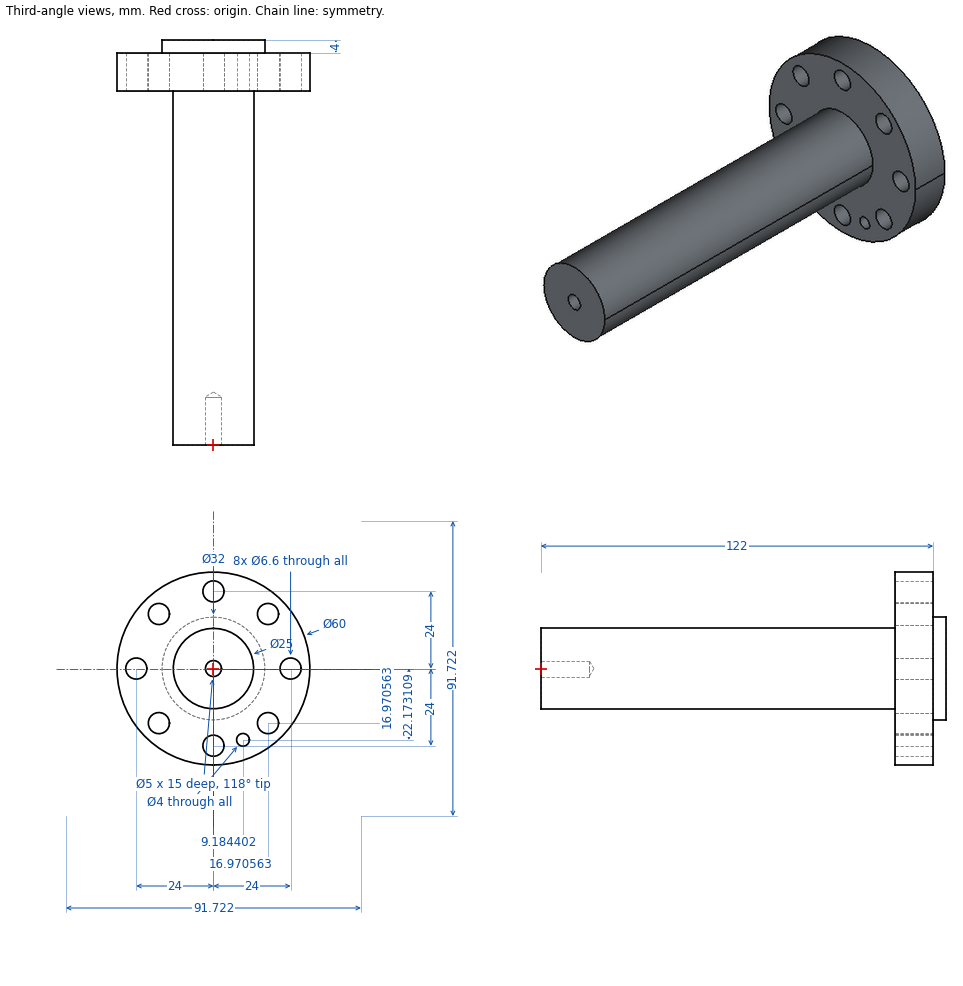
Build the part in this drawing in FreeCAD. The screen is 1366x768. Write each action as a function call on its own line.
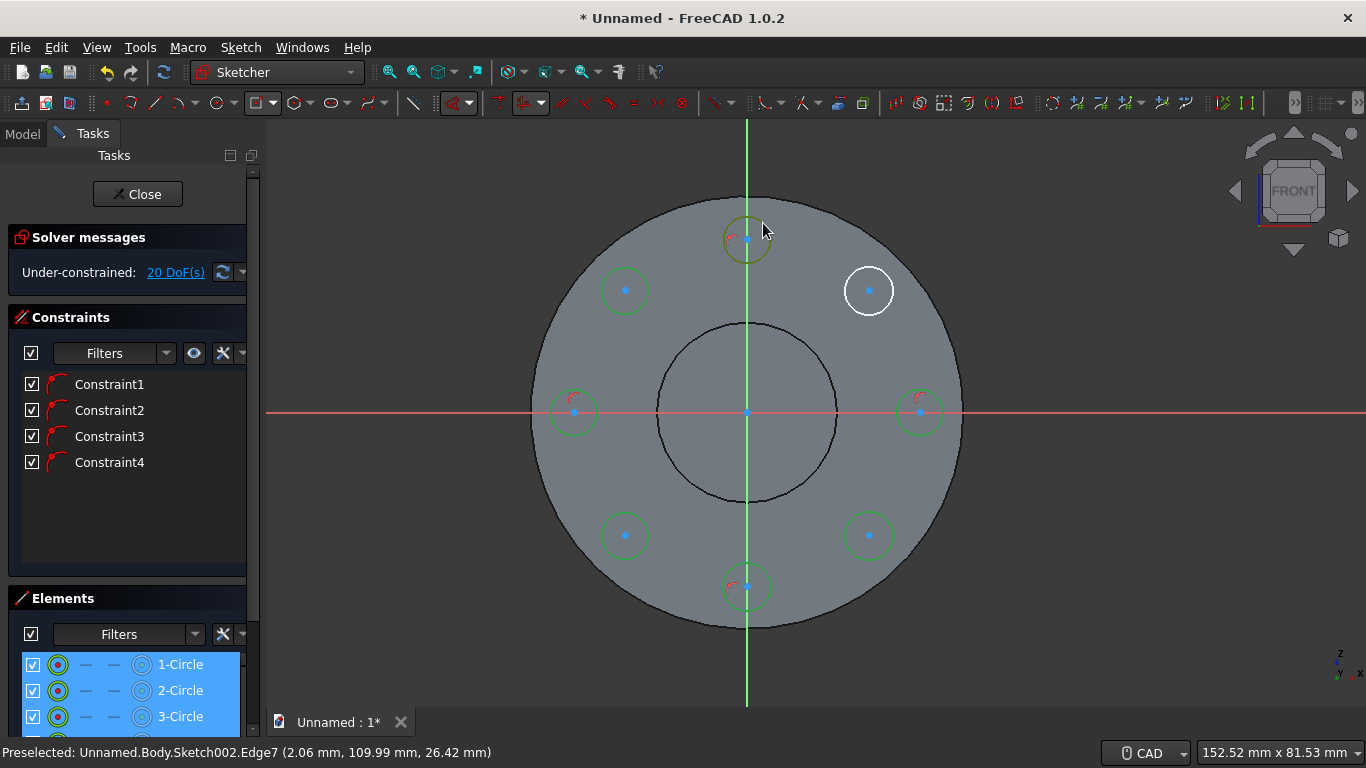
click(886, 274)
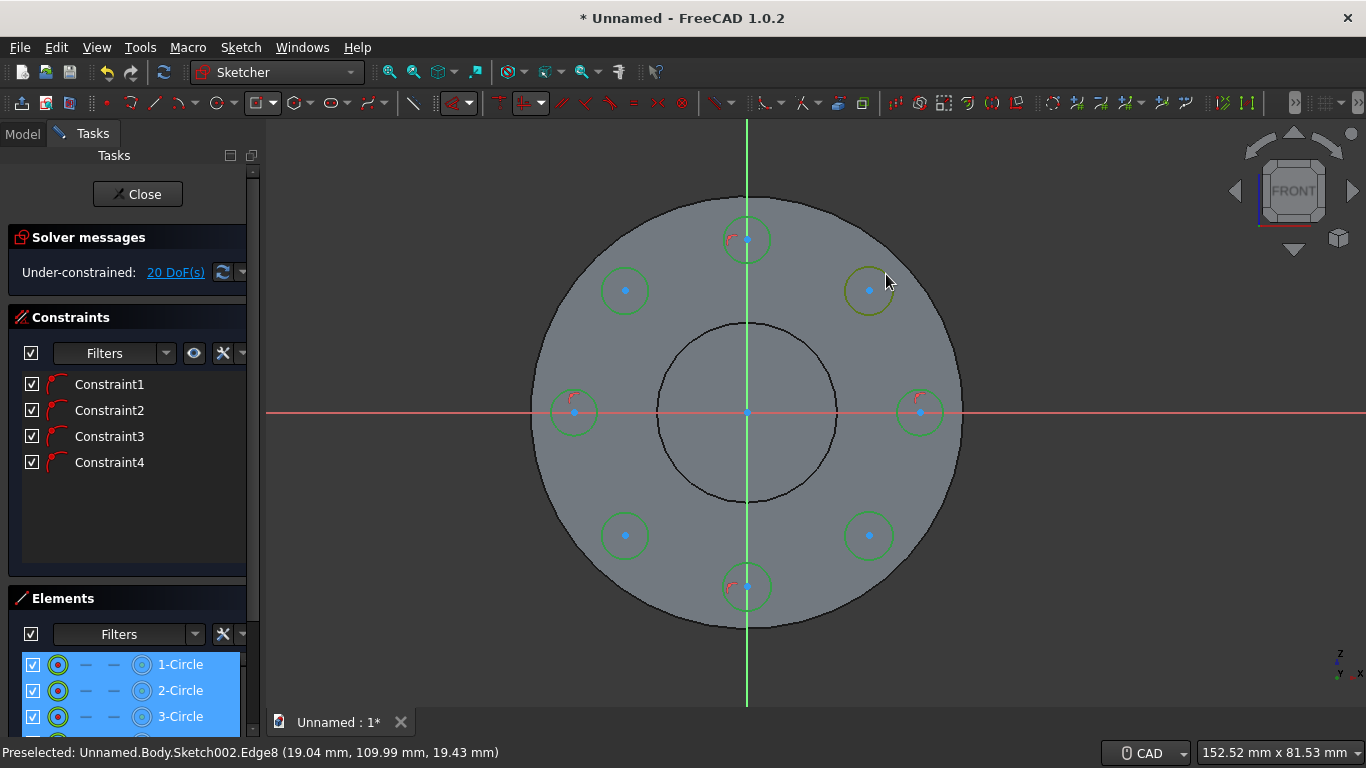
click(634, 104)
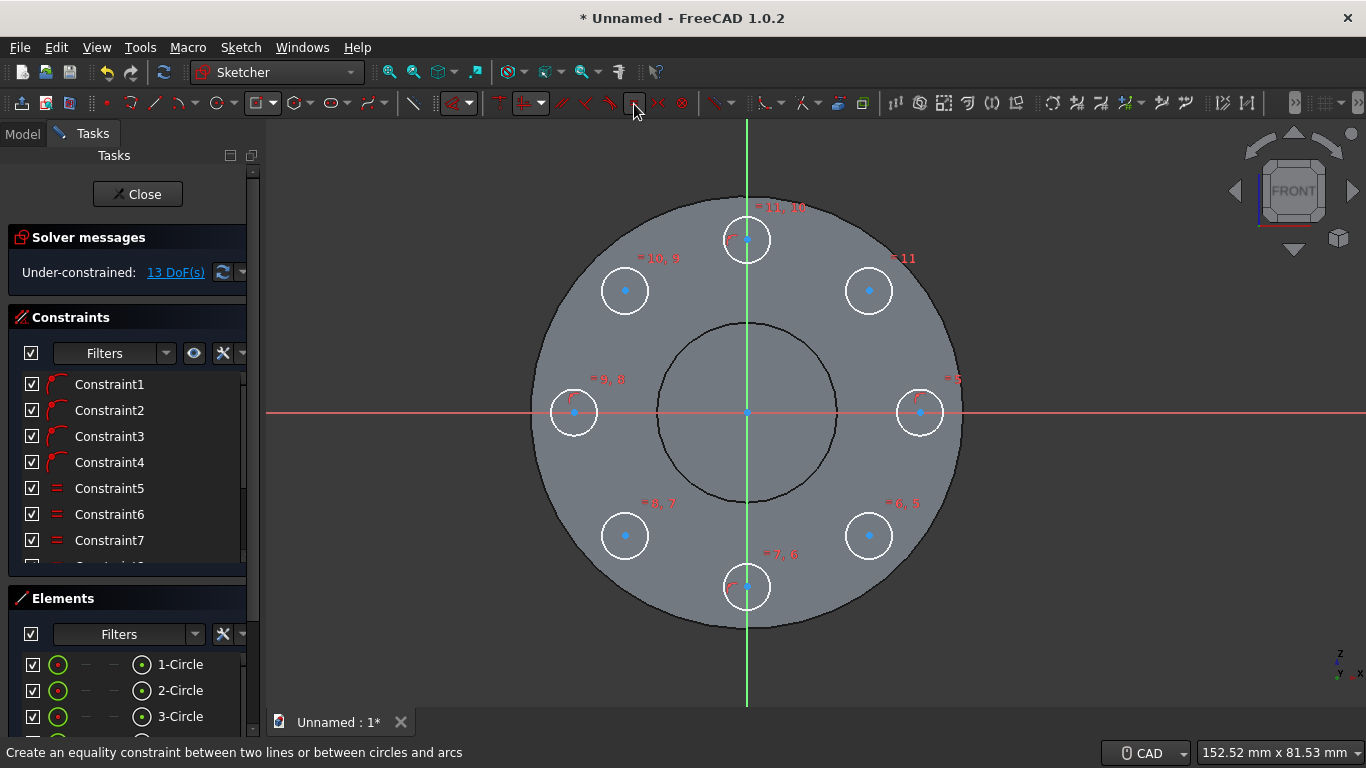
click(869, 536)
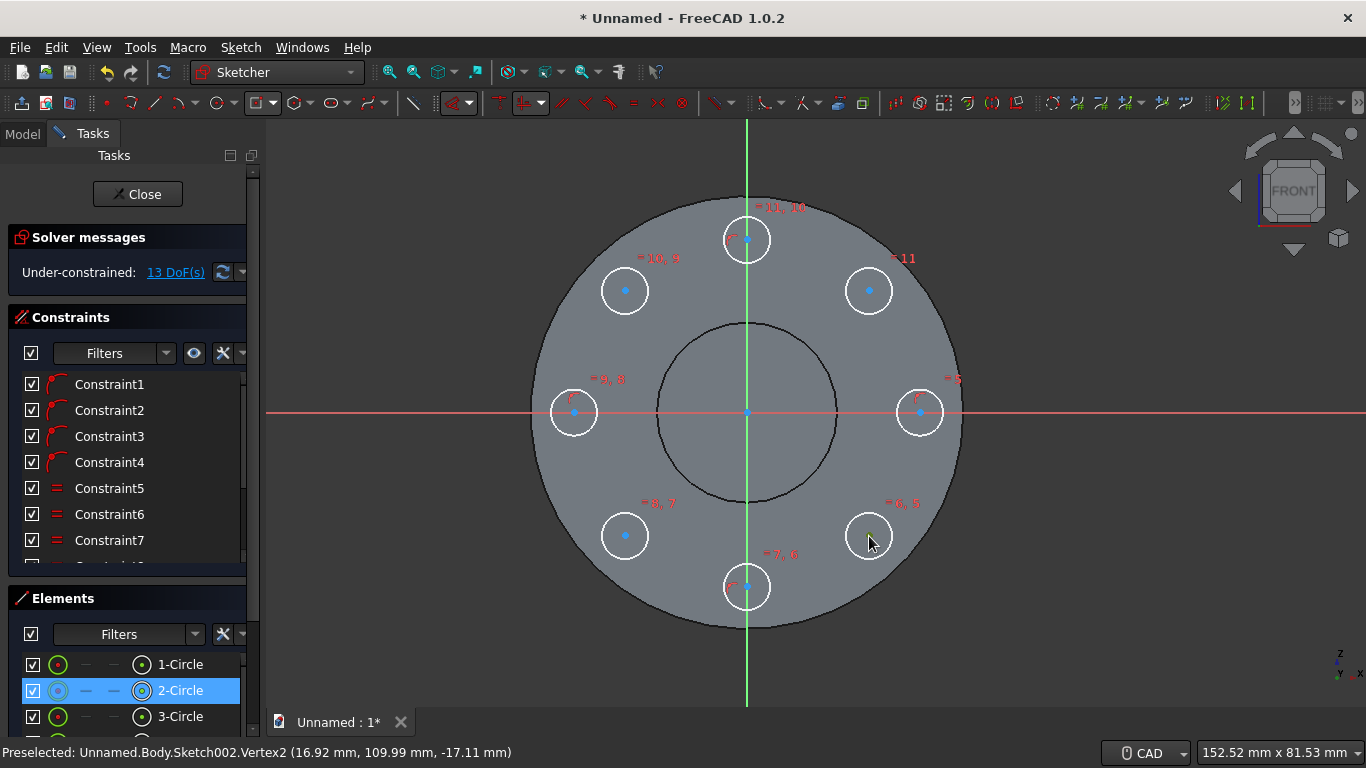
click(625, 536)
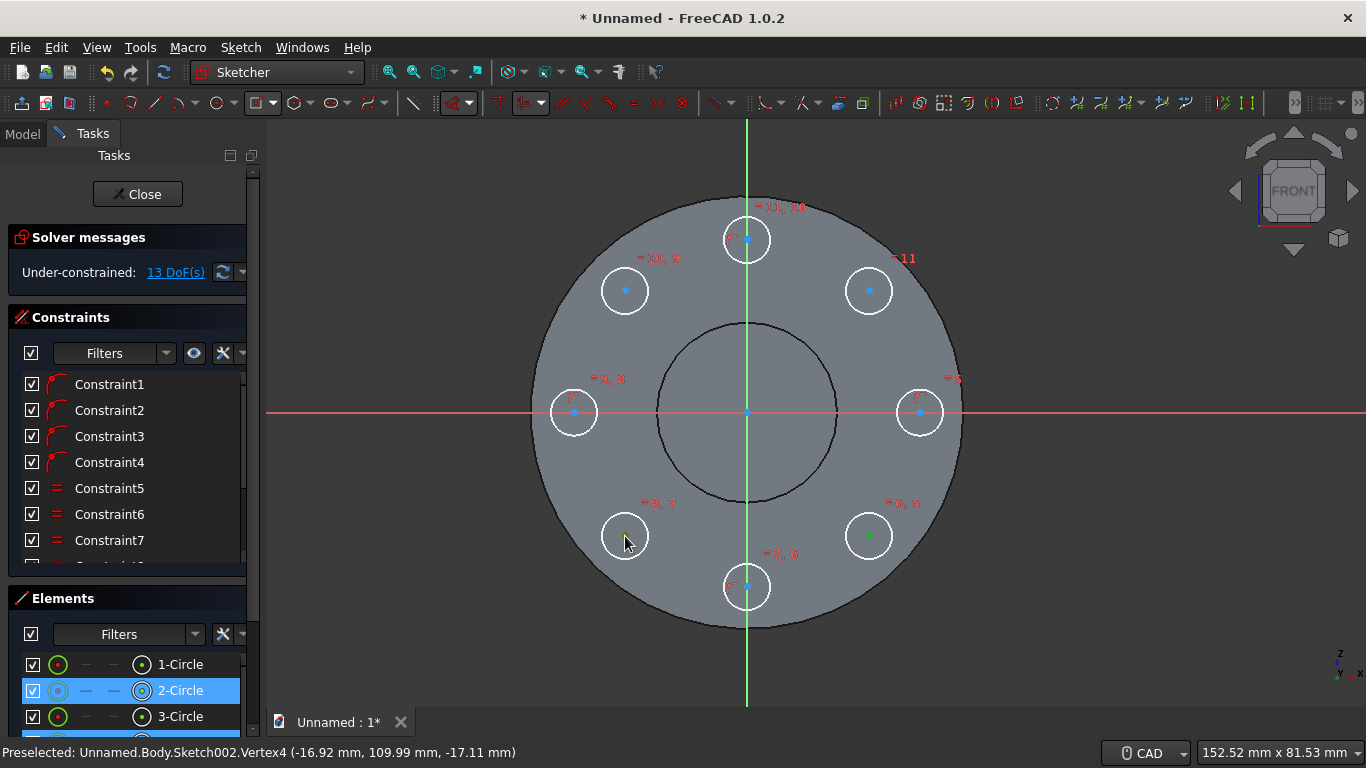
click(747, 641)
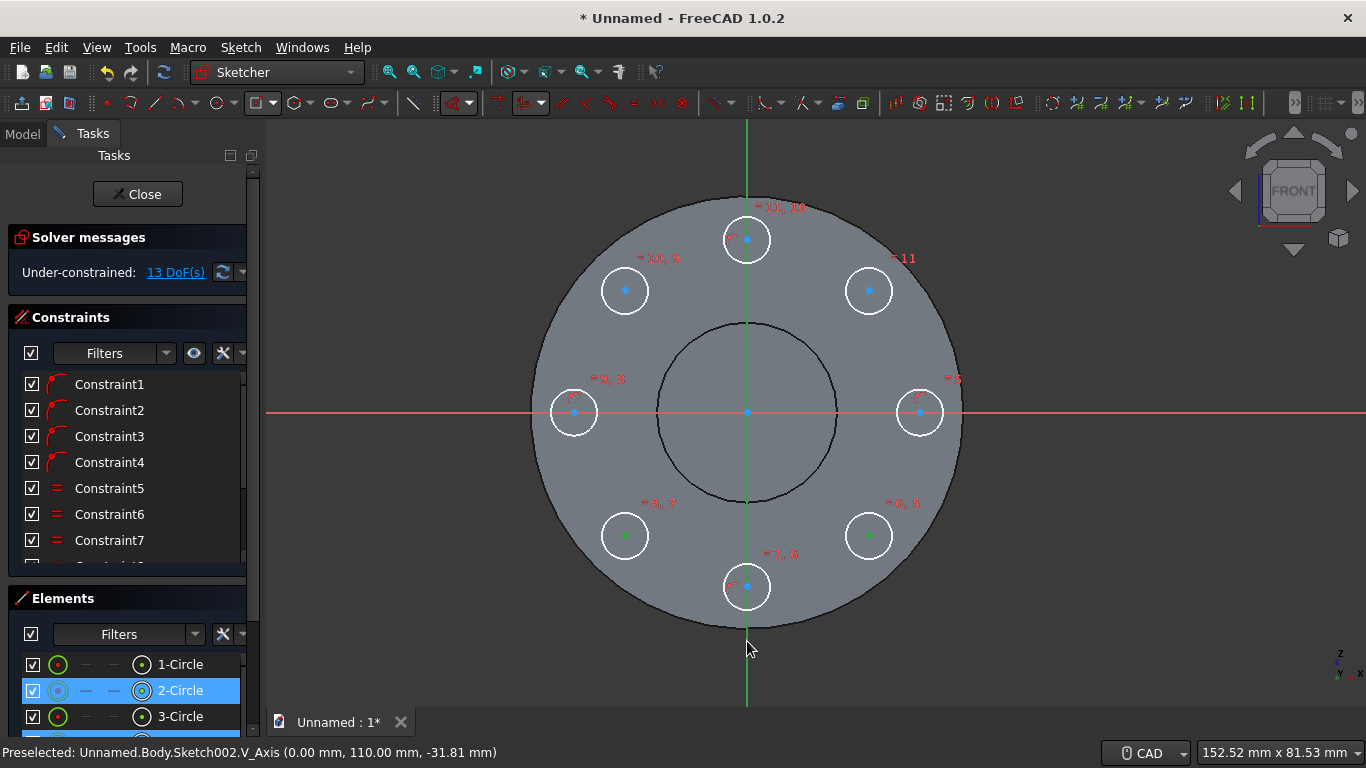
key(s)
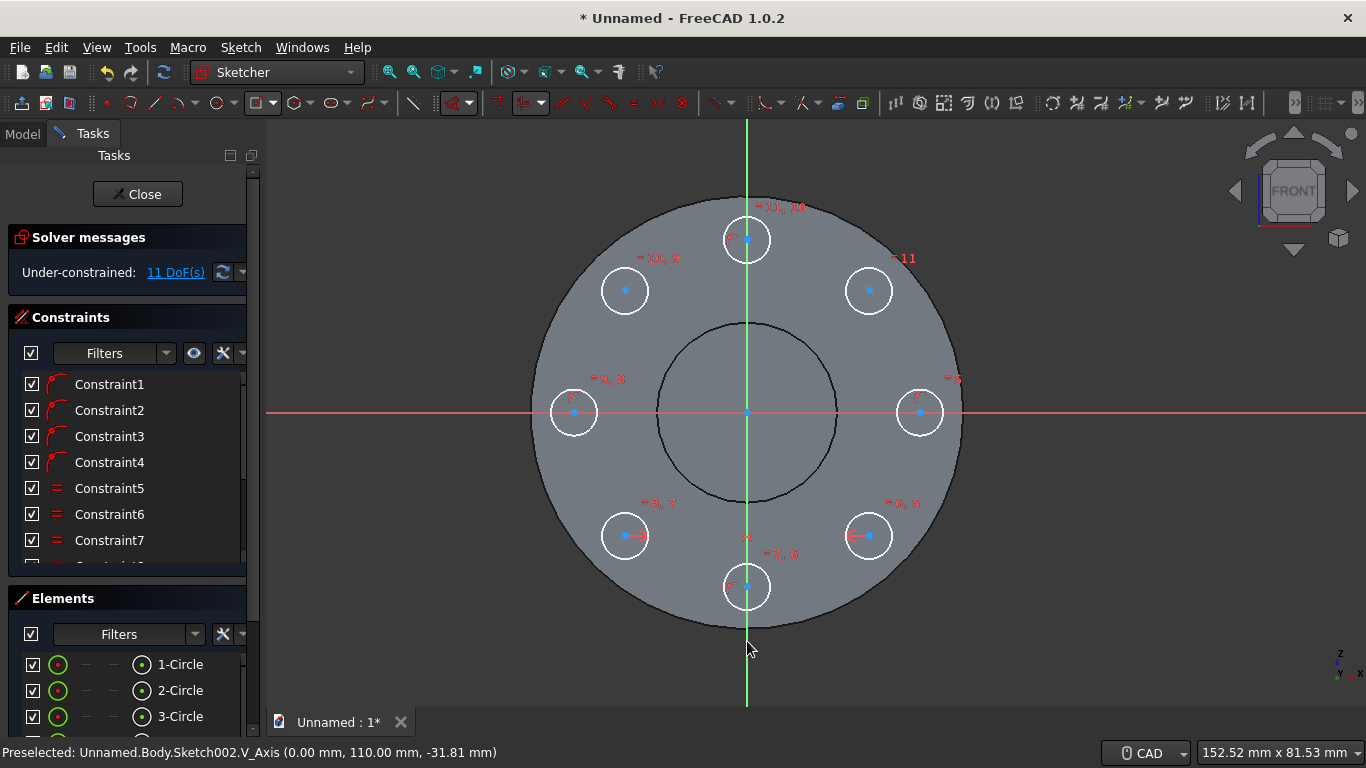
click(625, 536)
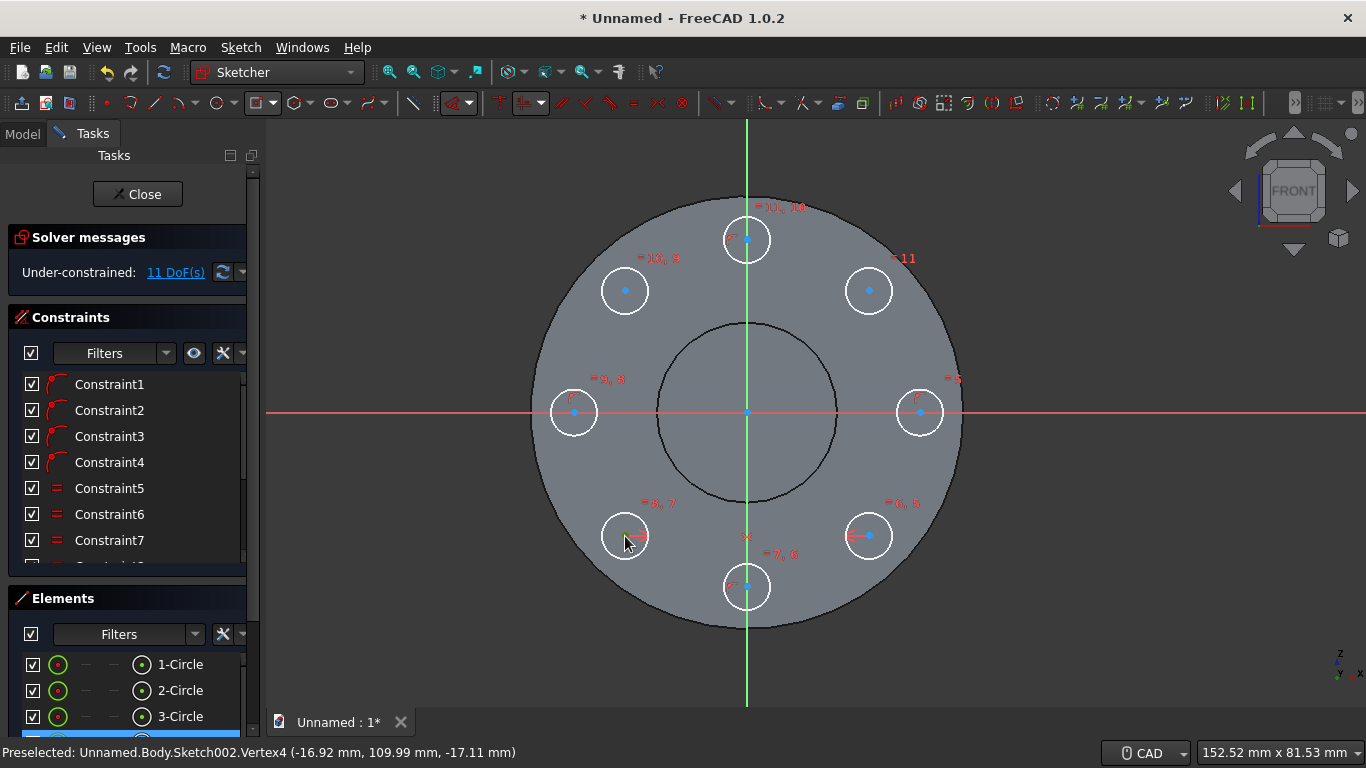
click(625, 291)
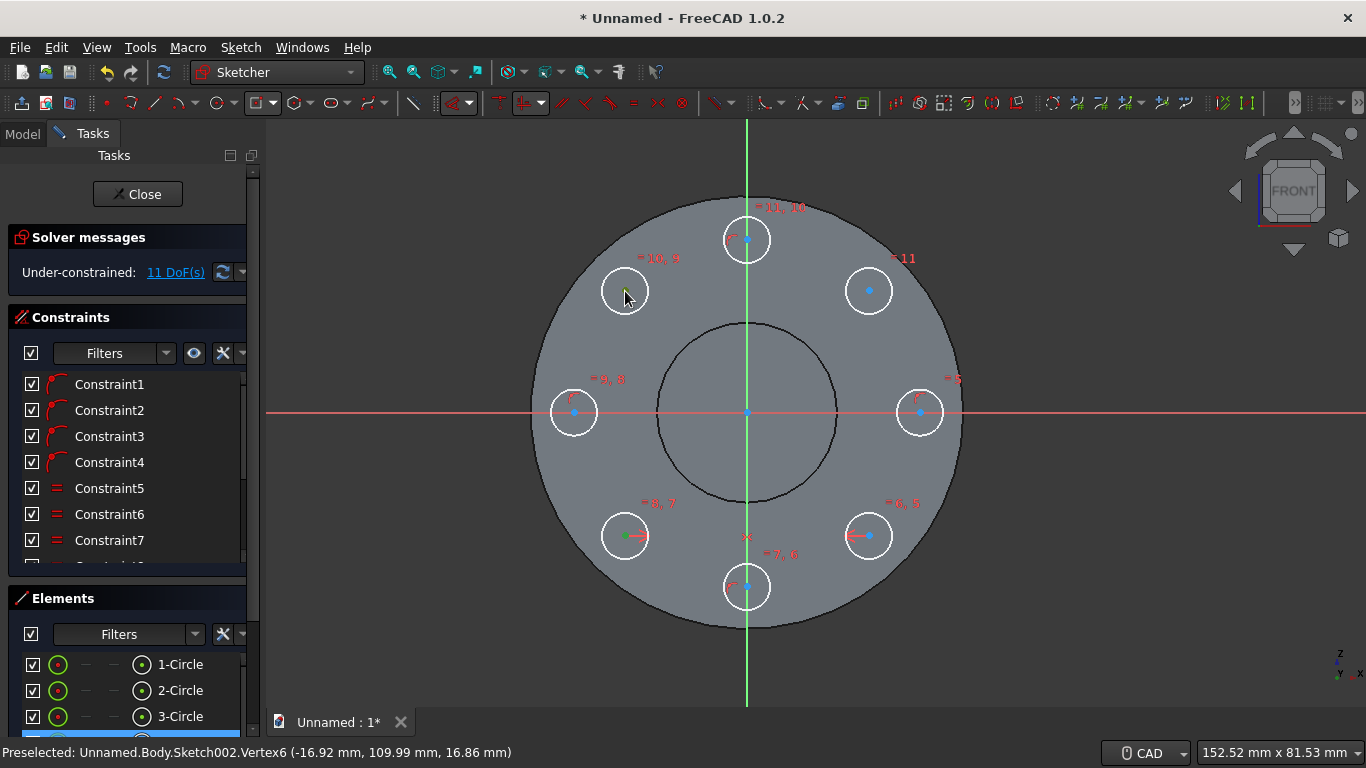
click(359, 413)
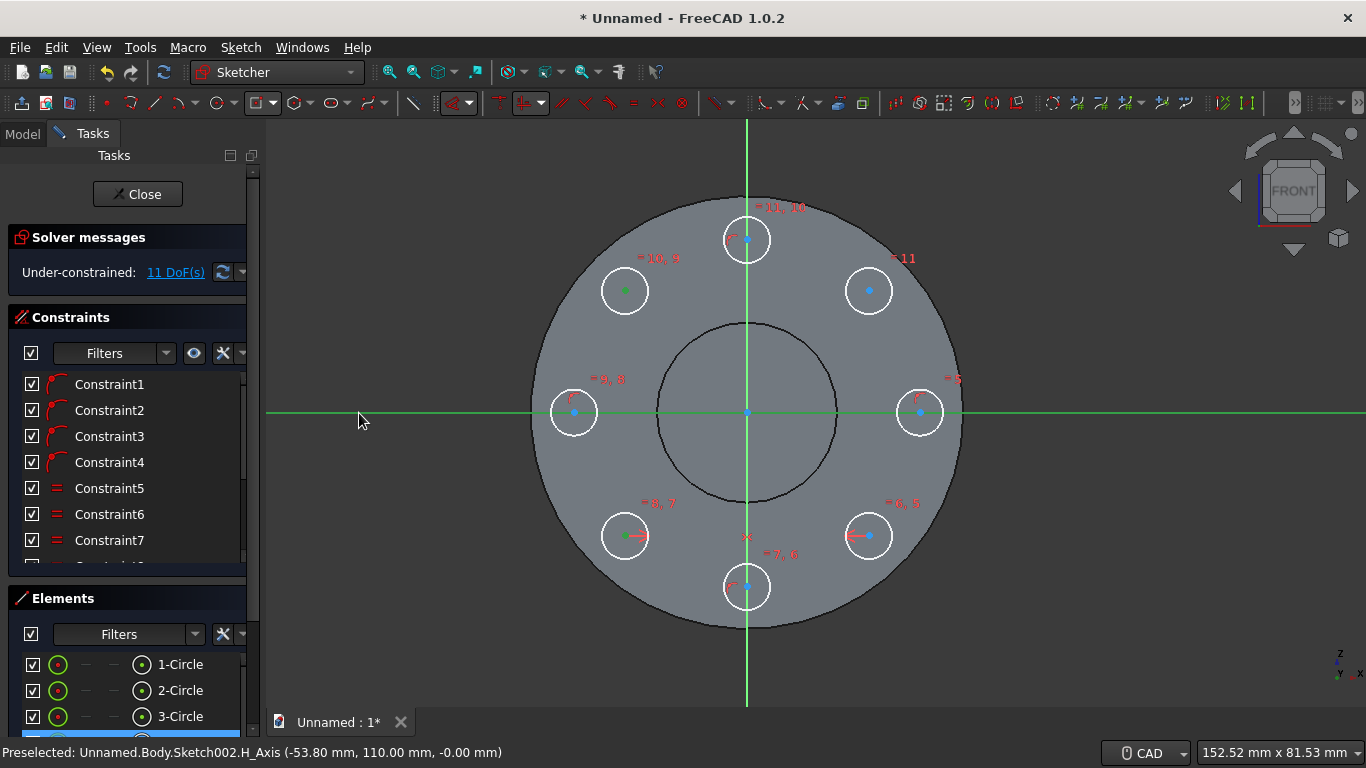
key(s)